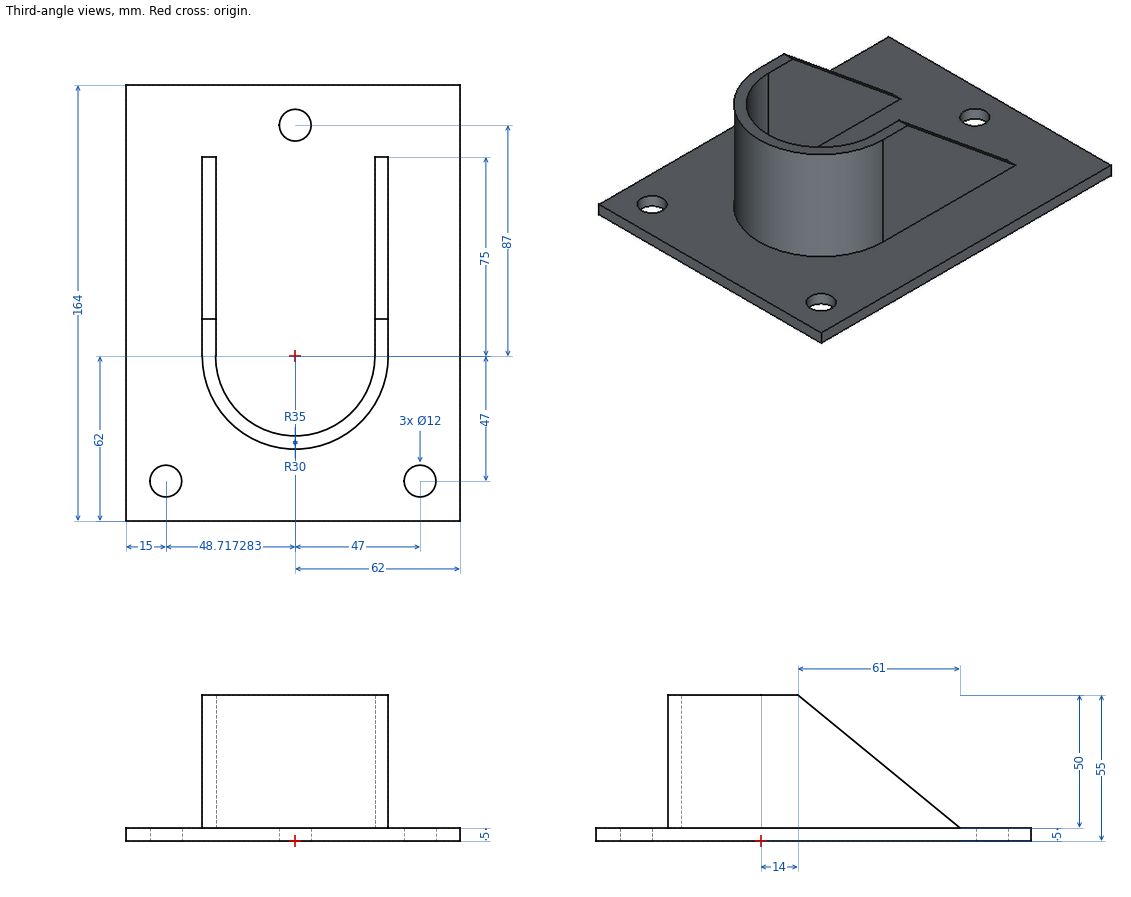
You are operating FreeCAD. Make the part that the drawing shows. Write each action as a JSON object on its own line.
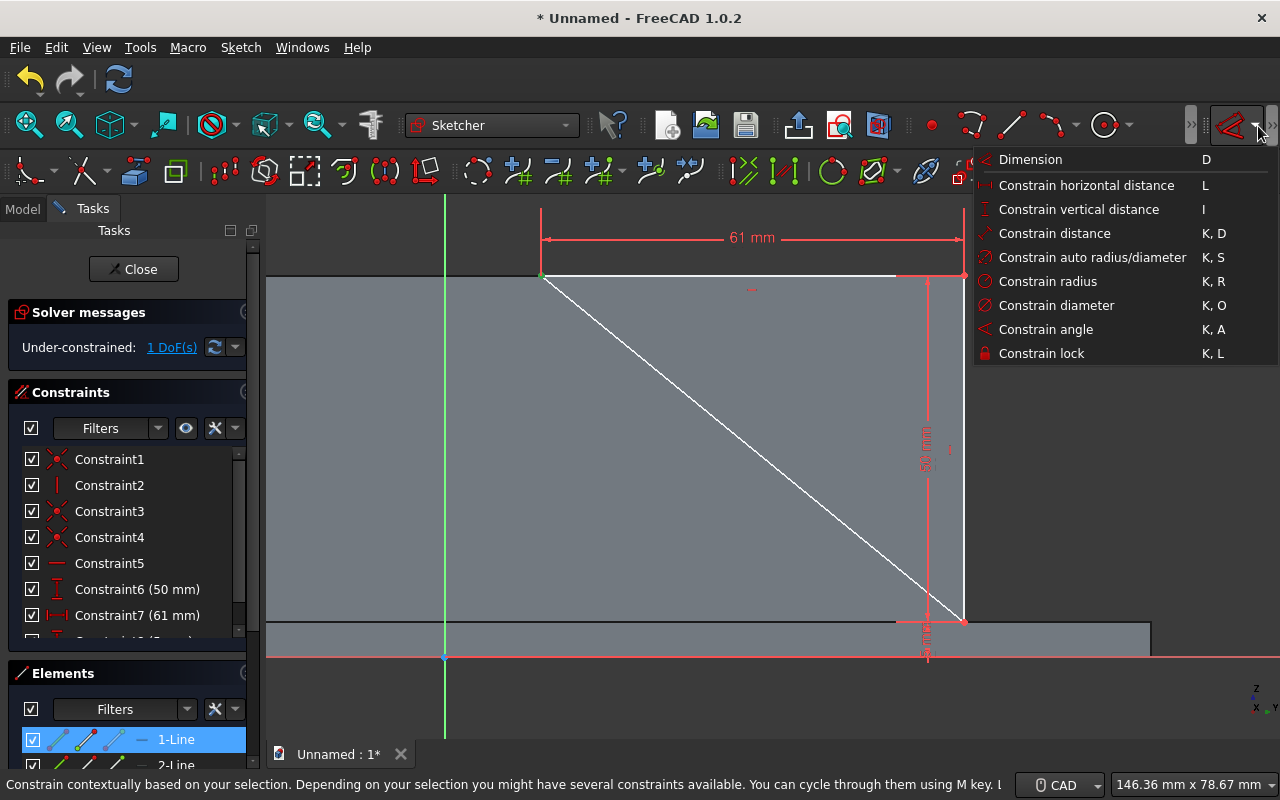
{"action": "left_click", "coordinate": [1126, 185]}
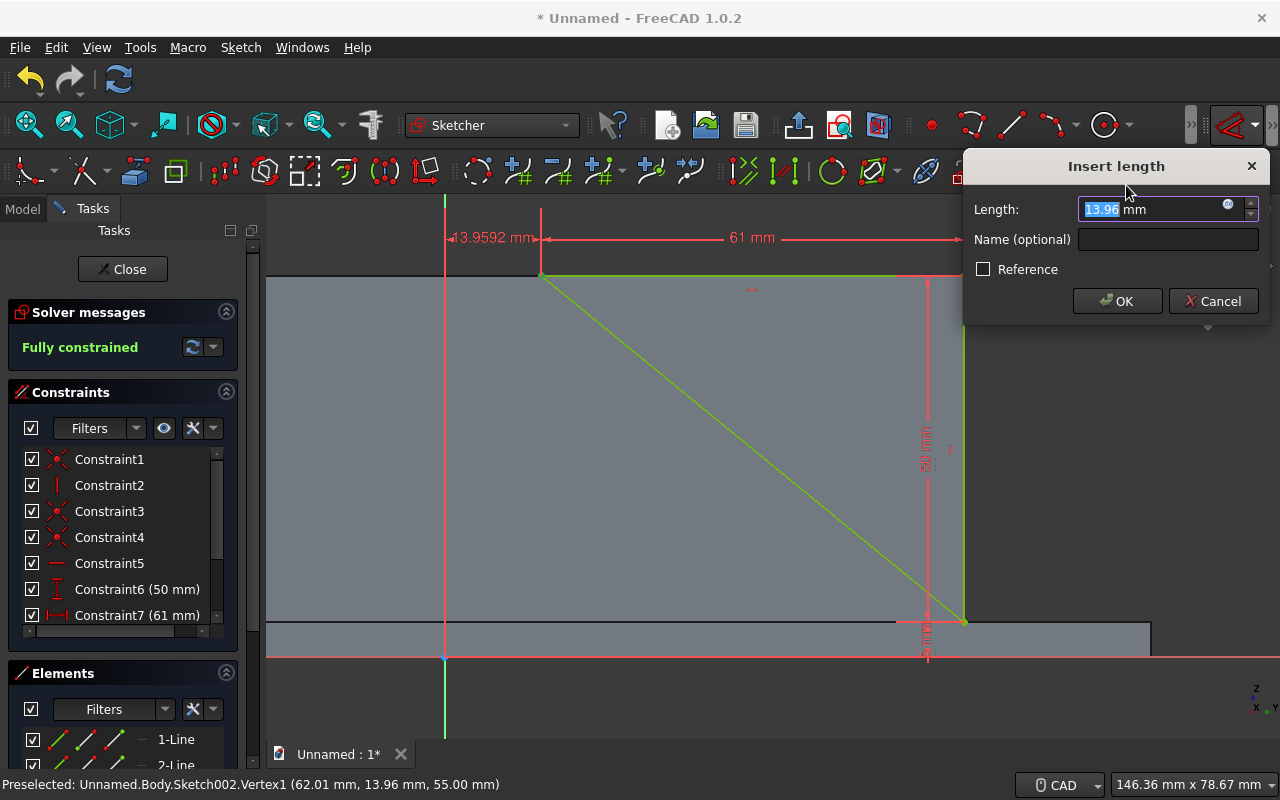
{"action": "type", "text": "14"}
{"action": "key", "text": "Return"}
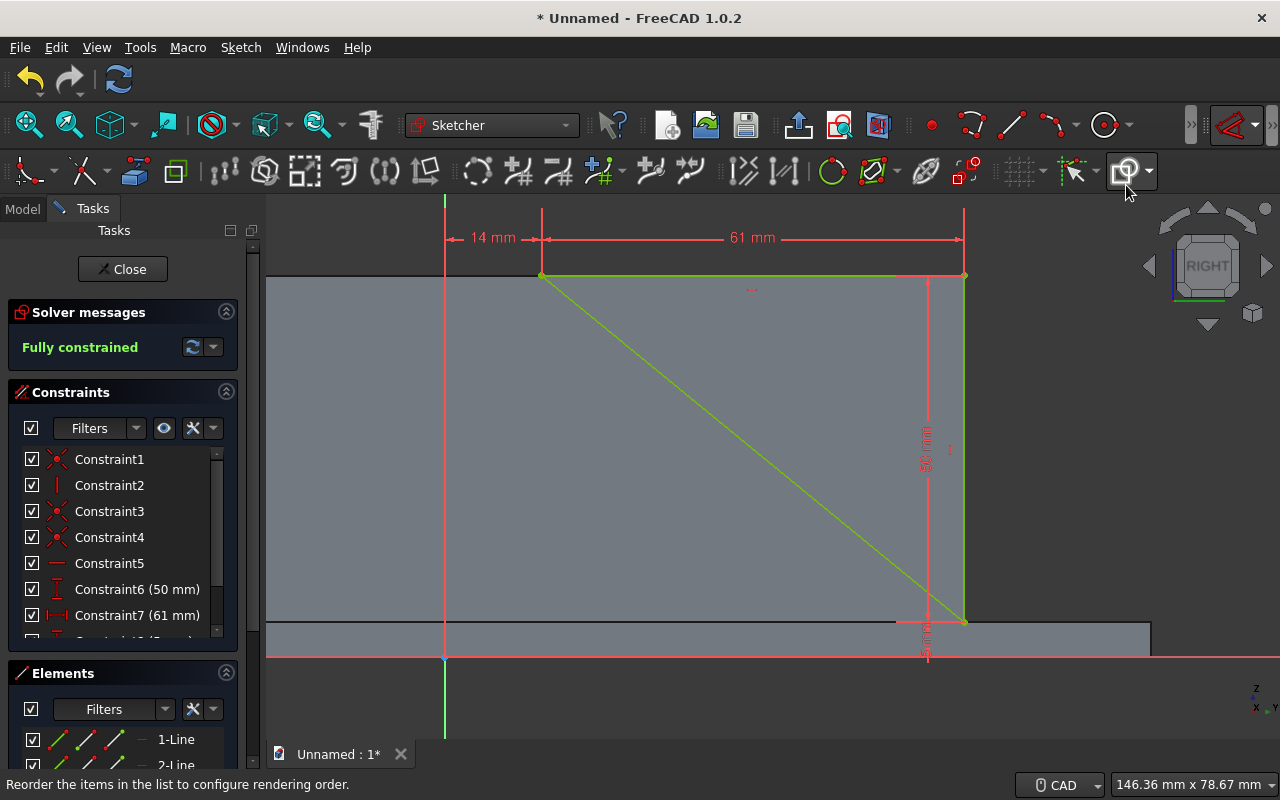
{"action": "left_click", "coordinate": [123, 269]}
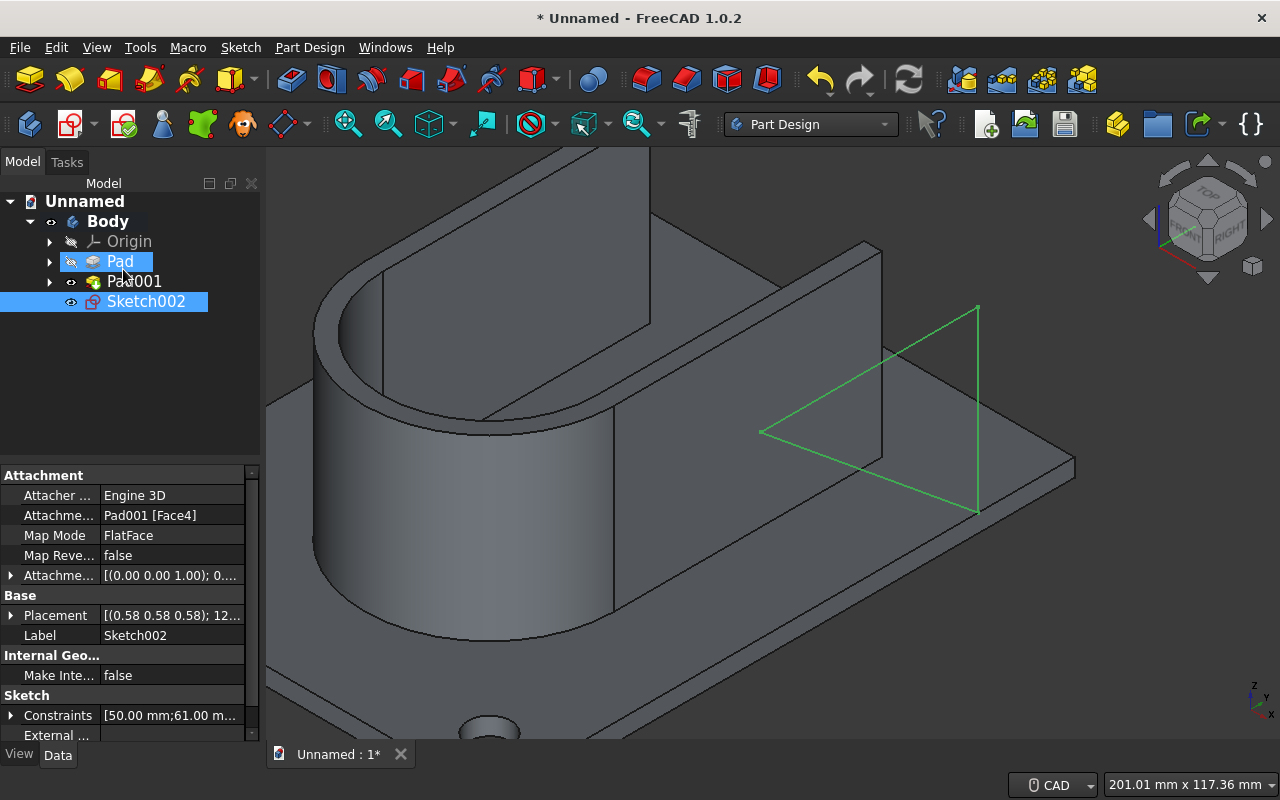
{"action": "left_click", "coordinate": [292, 80]}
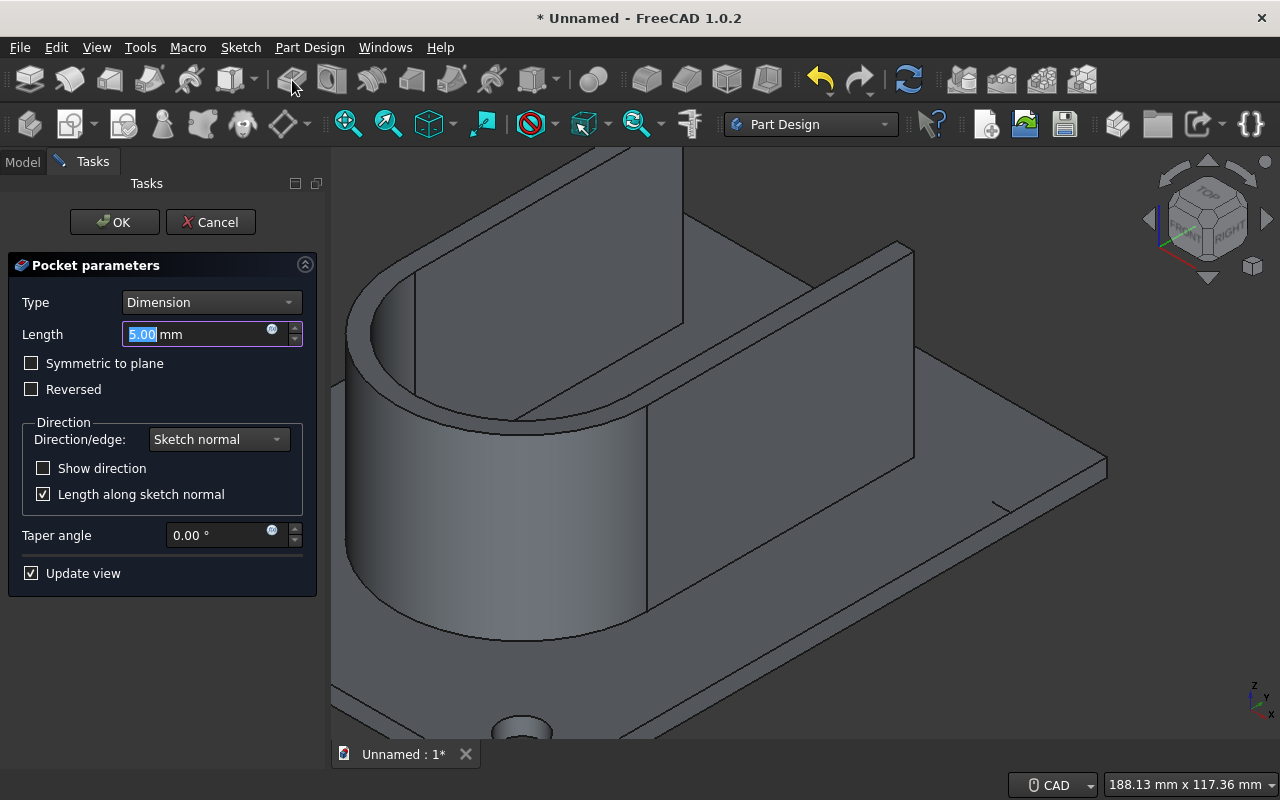
{"action": "left_click", "coordinate": [212, 302]}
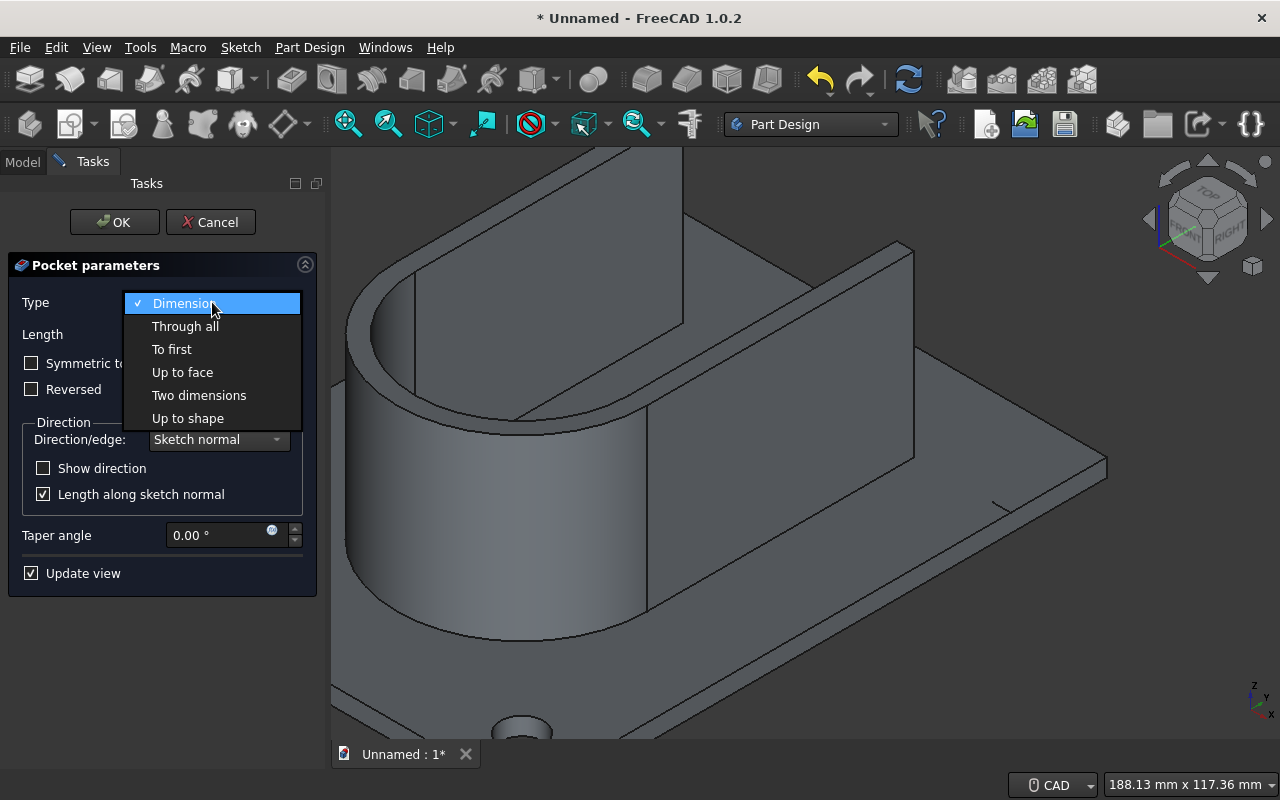
{"action": "left_click", "coordinate": [212, 326]}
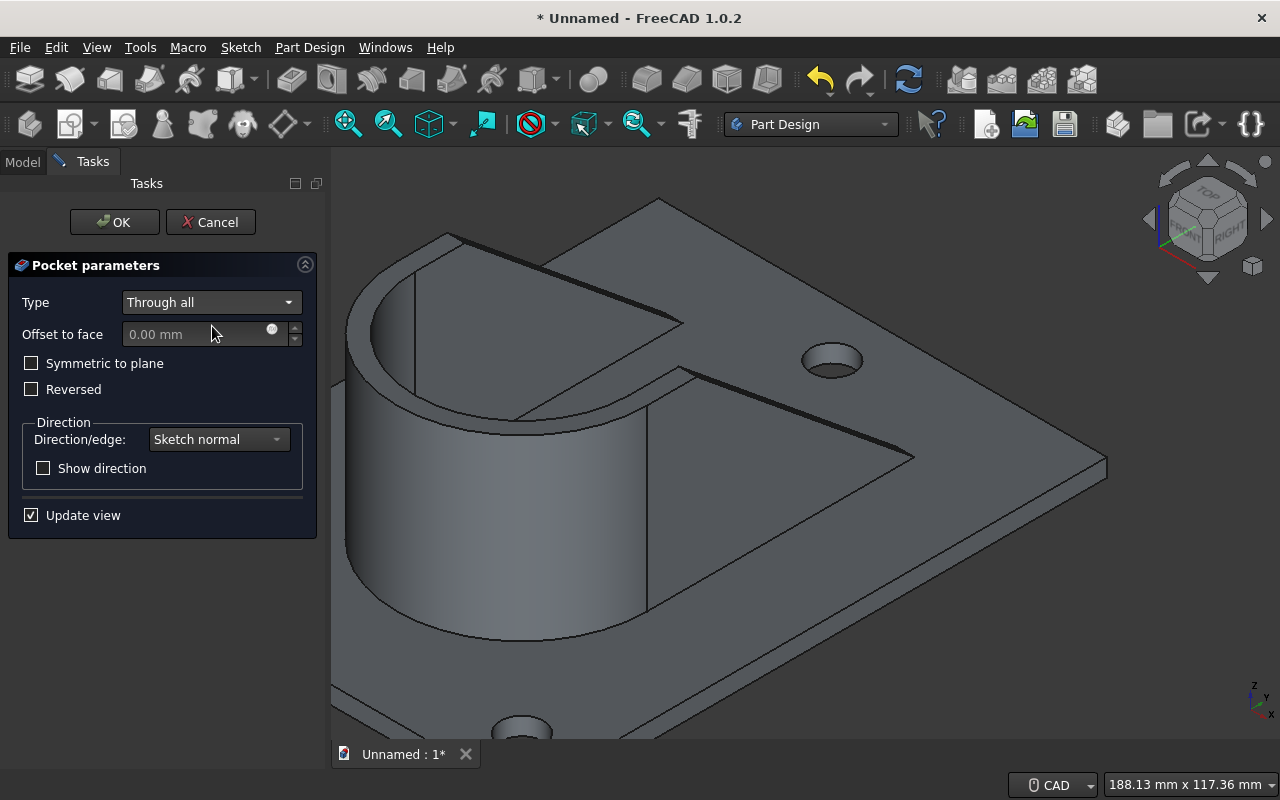
{"action": "left_click", "coordinate": [115, 222]}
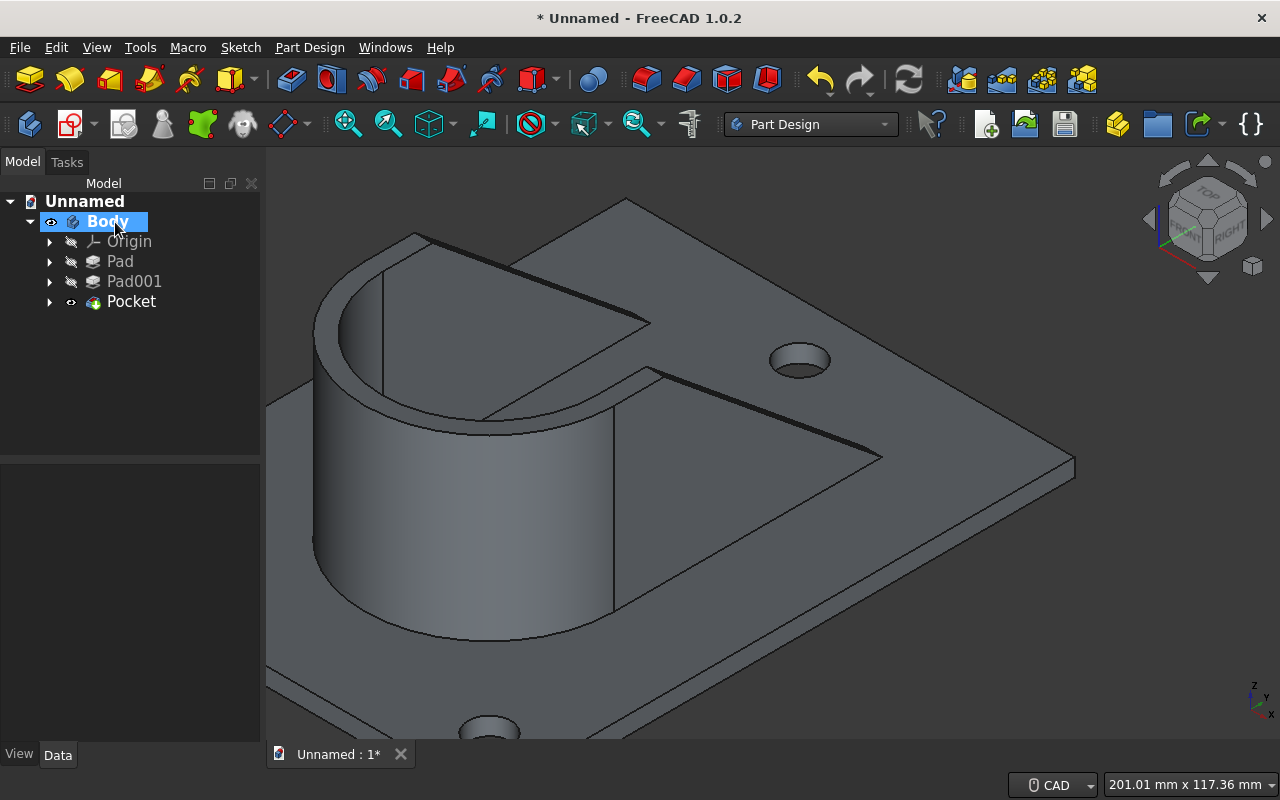
{"action": "left_click", "coordinate": [350, 124]}